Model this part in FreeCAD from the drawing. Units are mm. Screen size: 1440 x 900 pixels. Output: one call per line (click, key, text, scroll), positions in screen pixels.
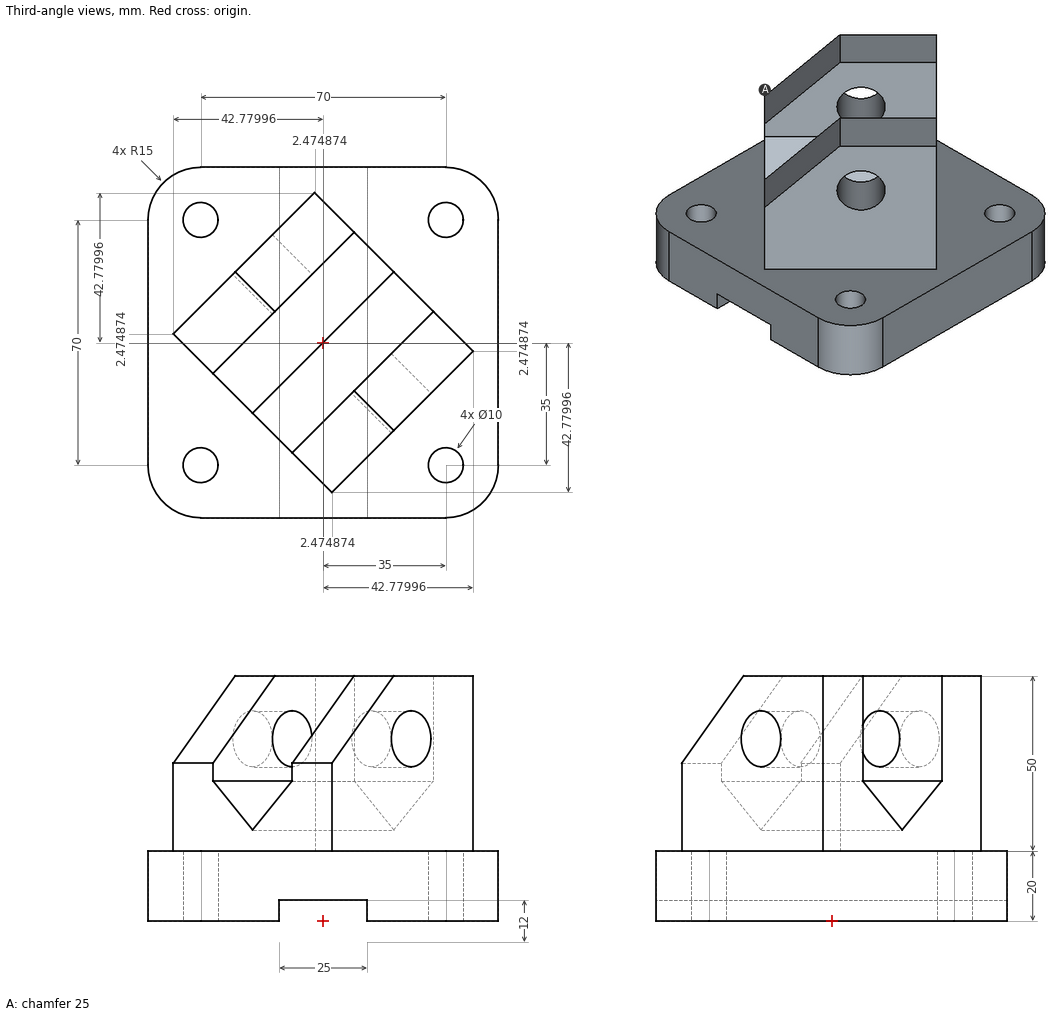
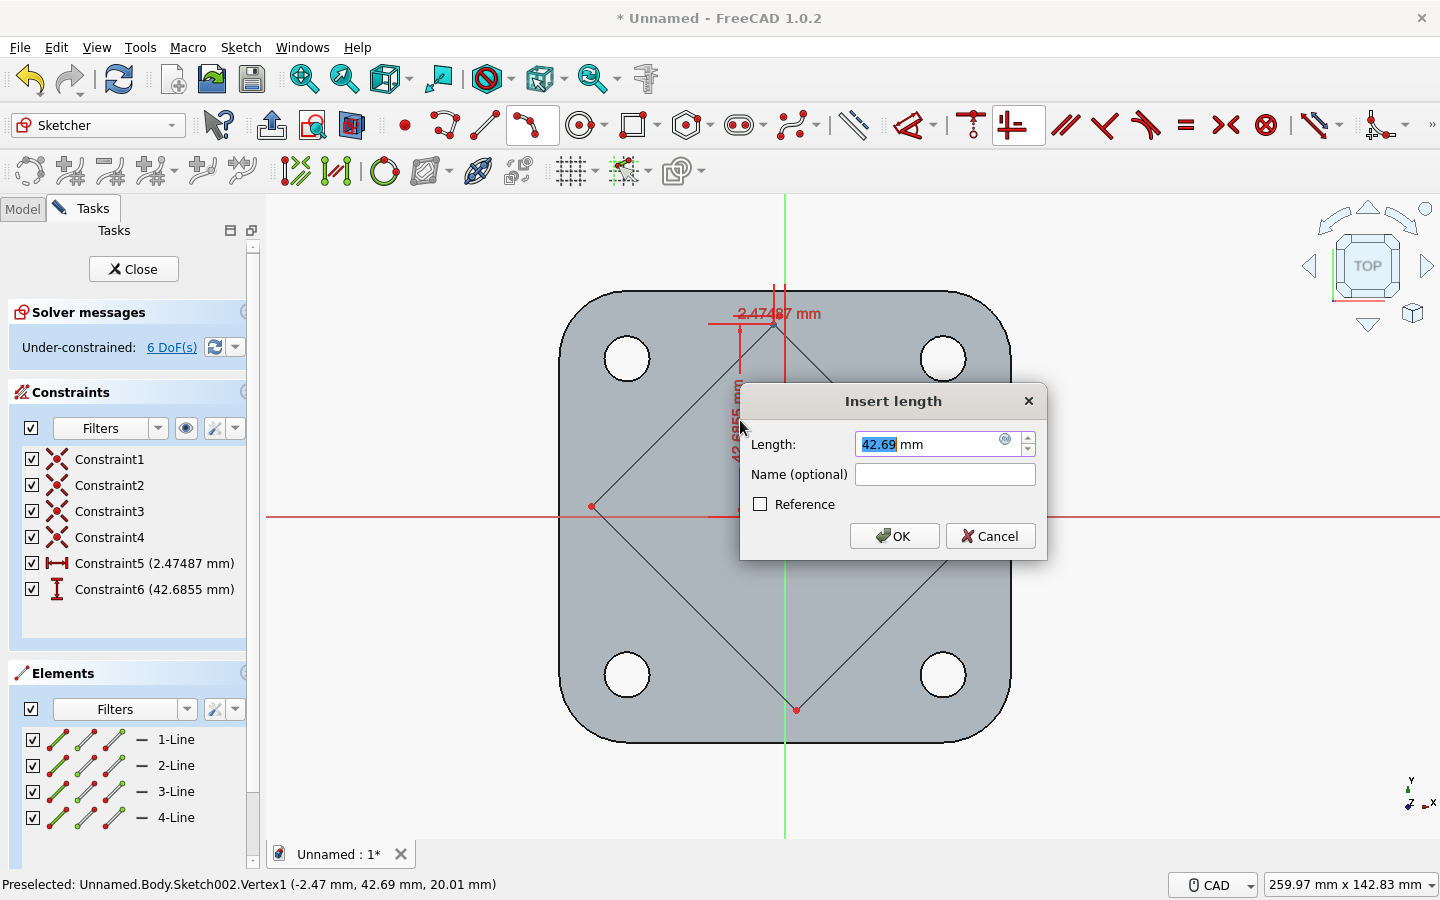
text(42.77996)
key(Return)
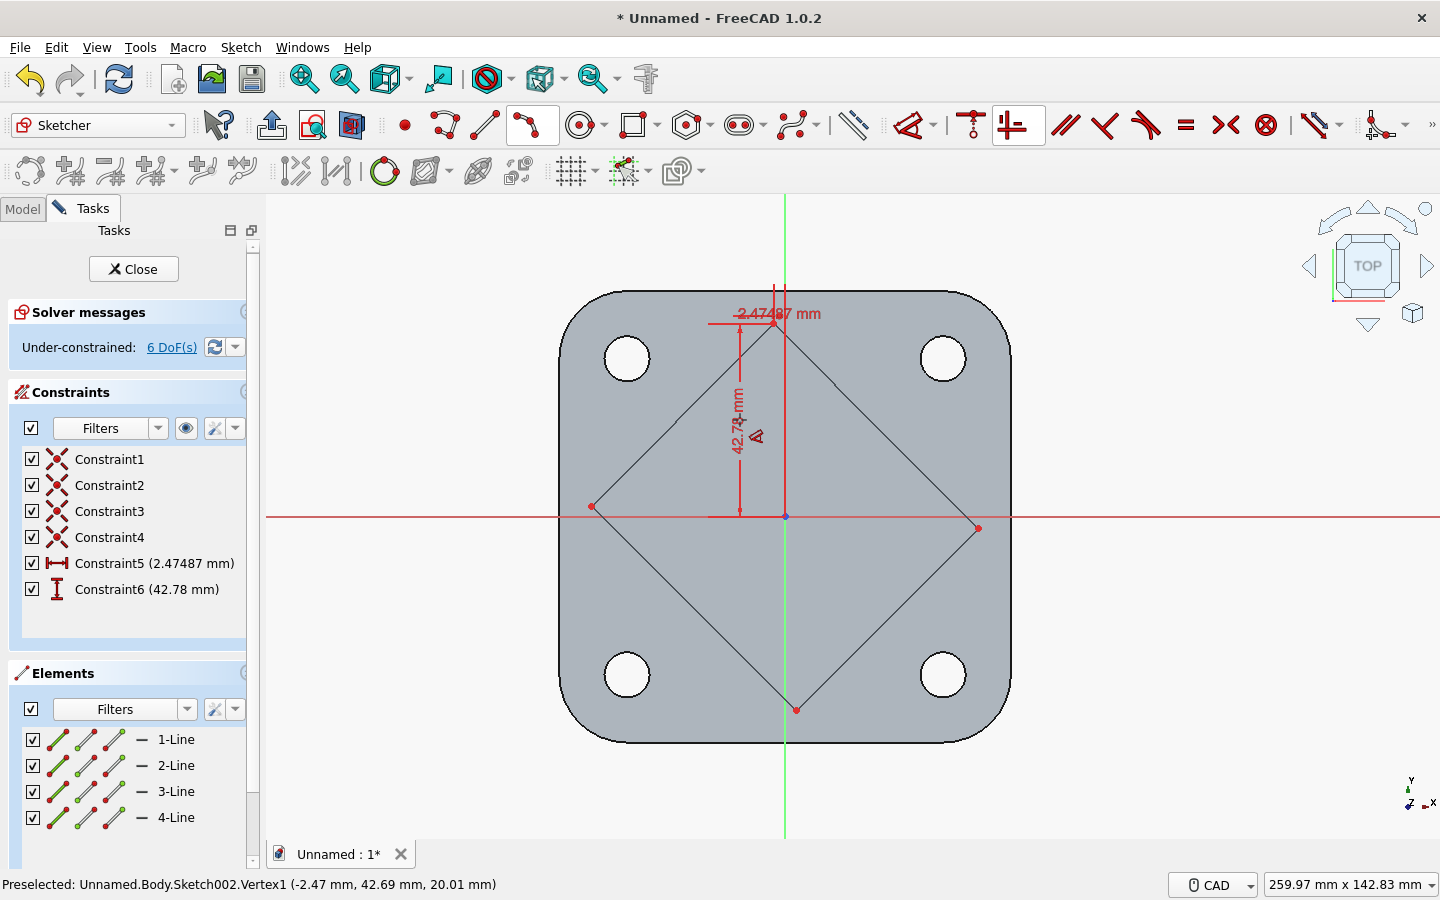
click(592, 506)
click(689, 472)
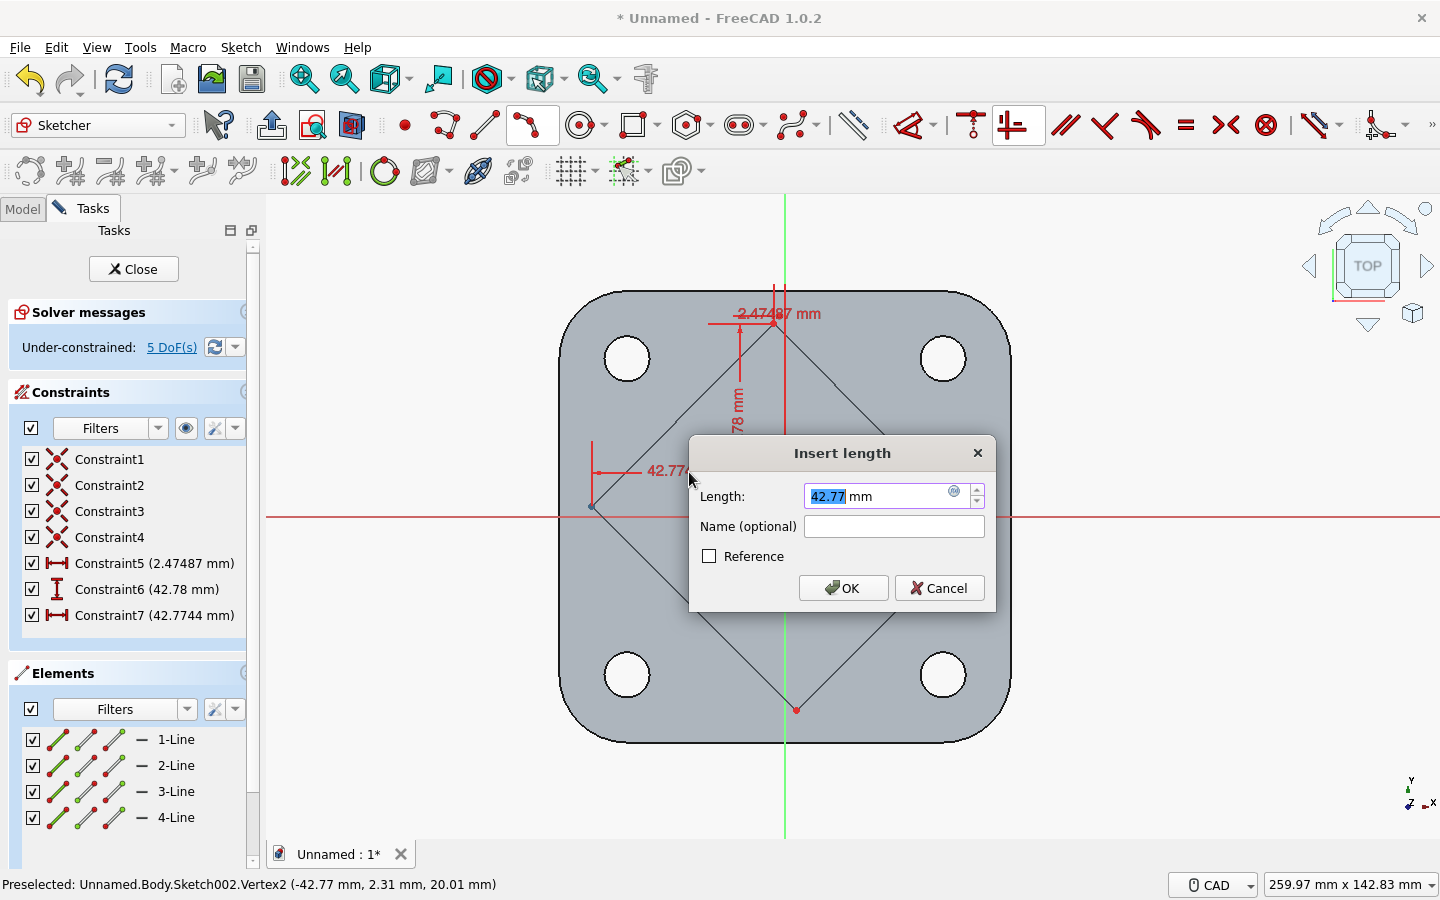
text(42.77996)
key(Return)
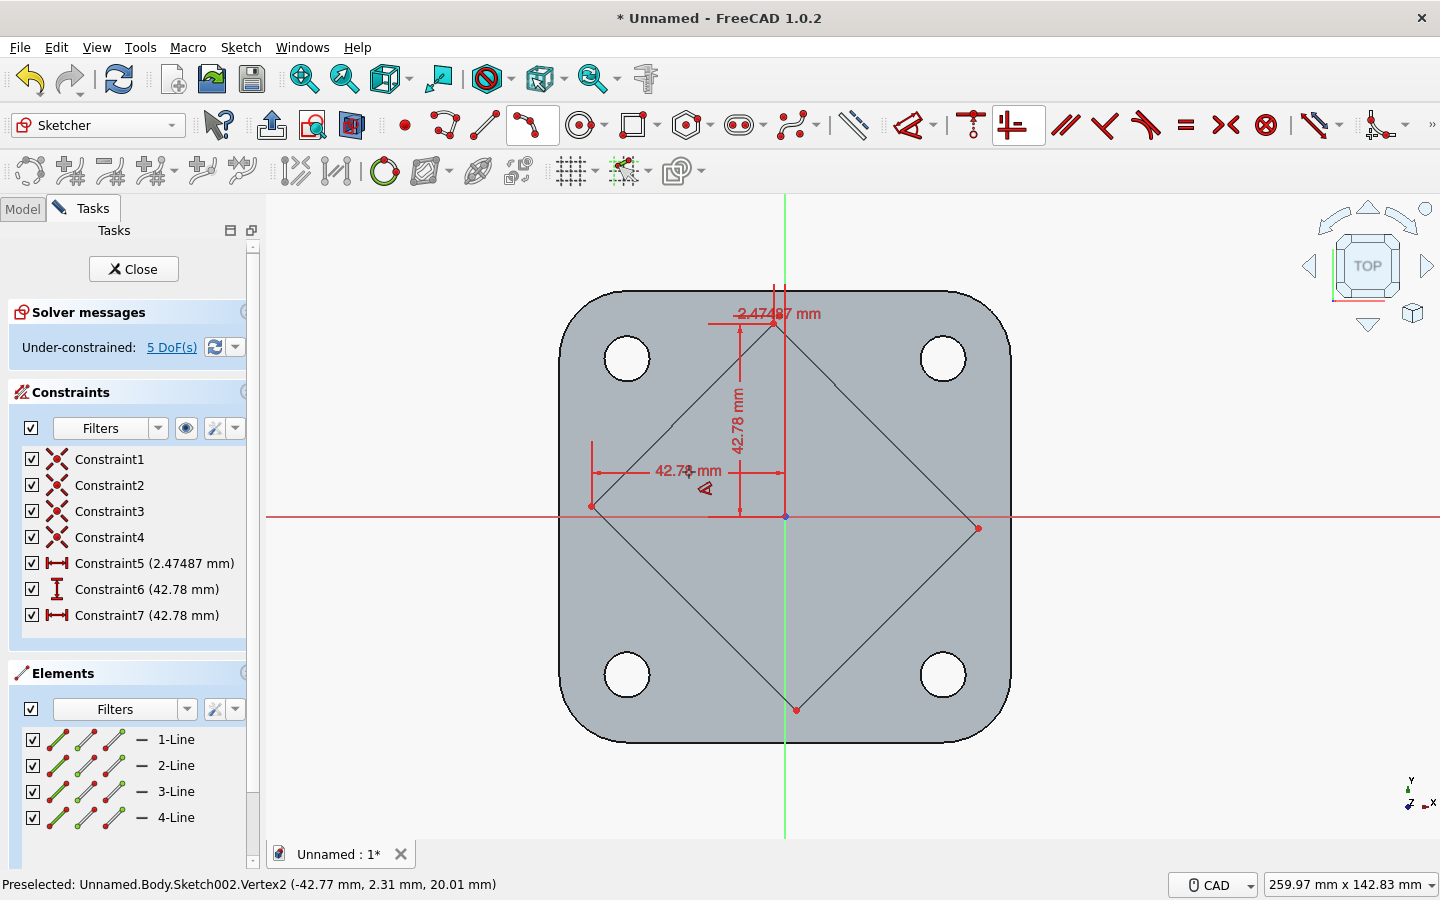
scroll(592, 506, up, 7)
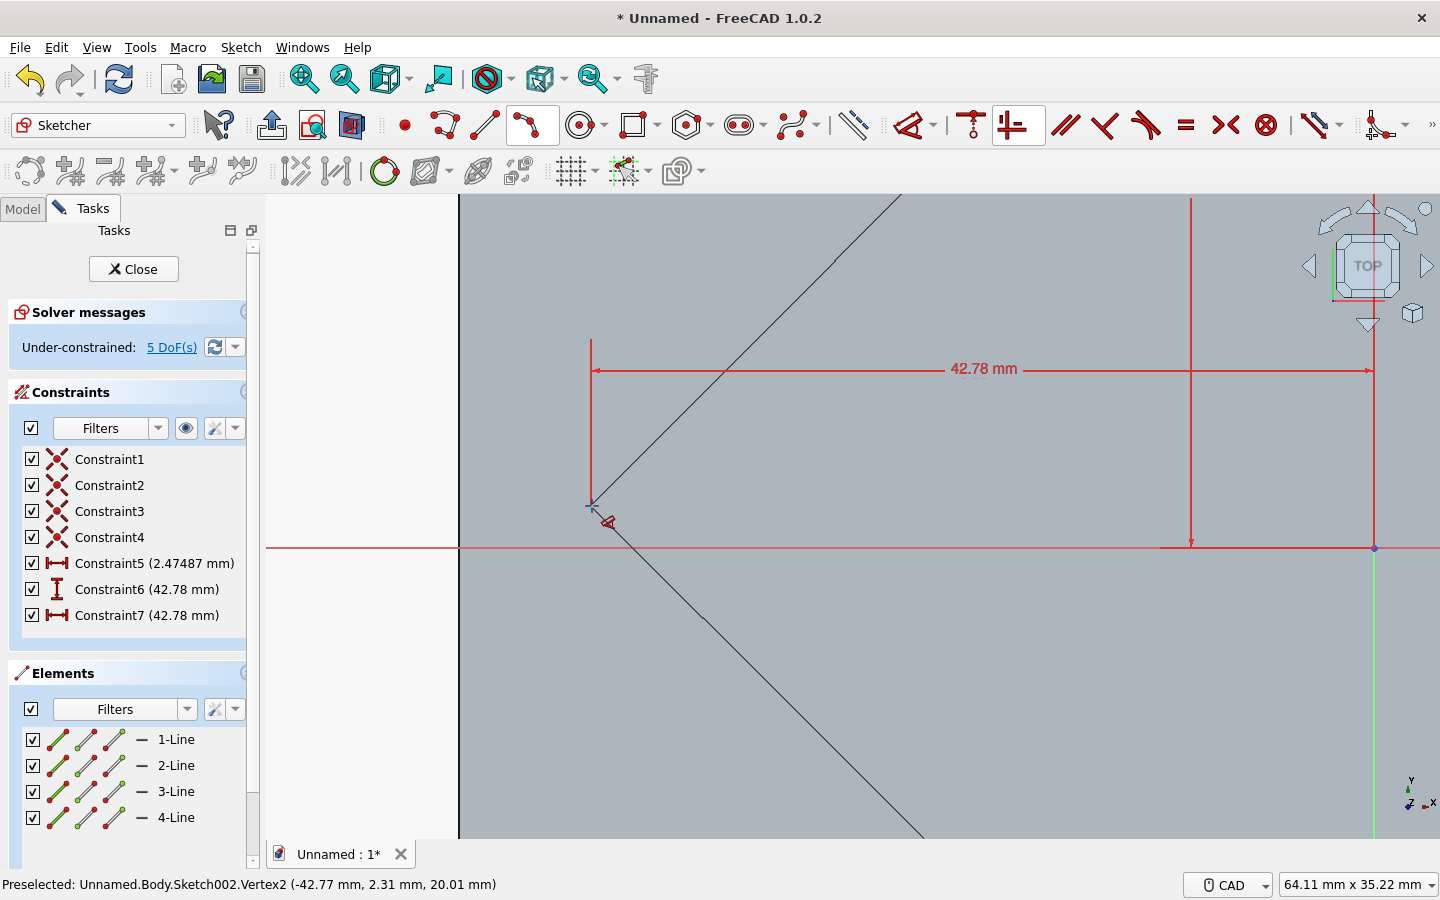
click(591, 506)
click(557, 527)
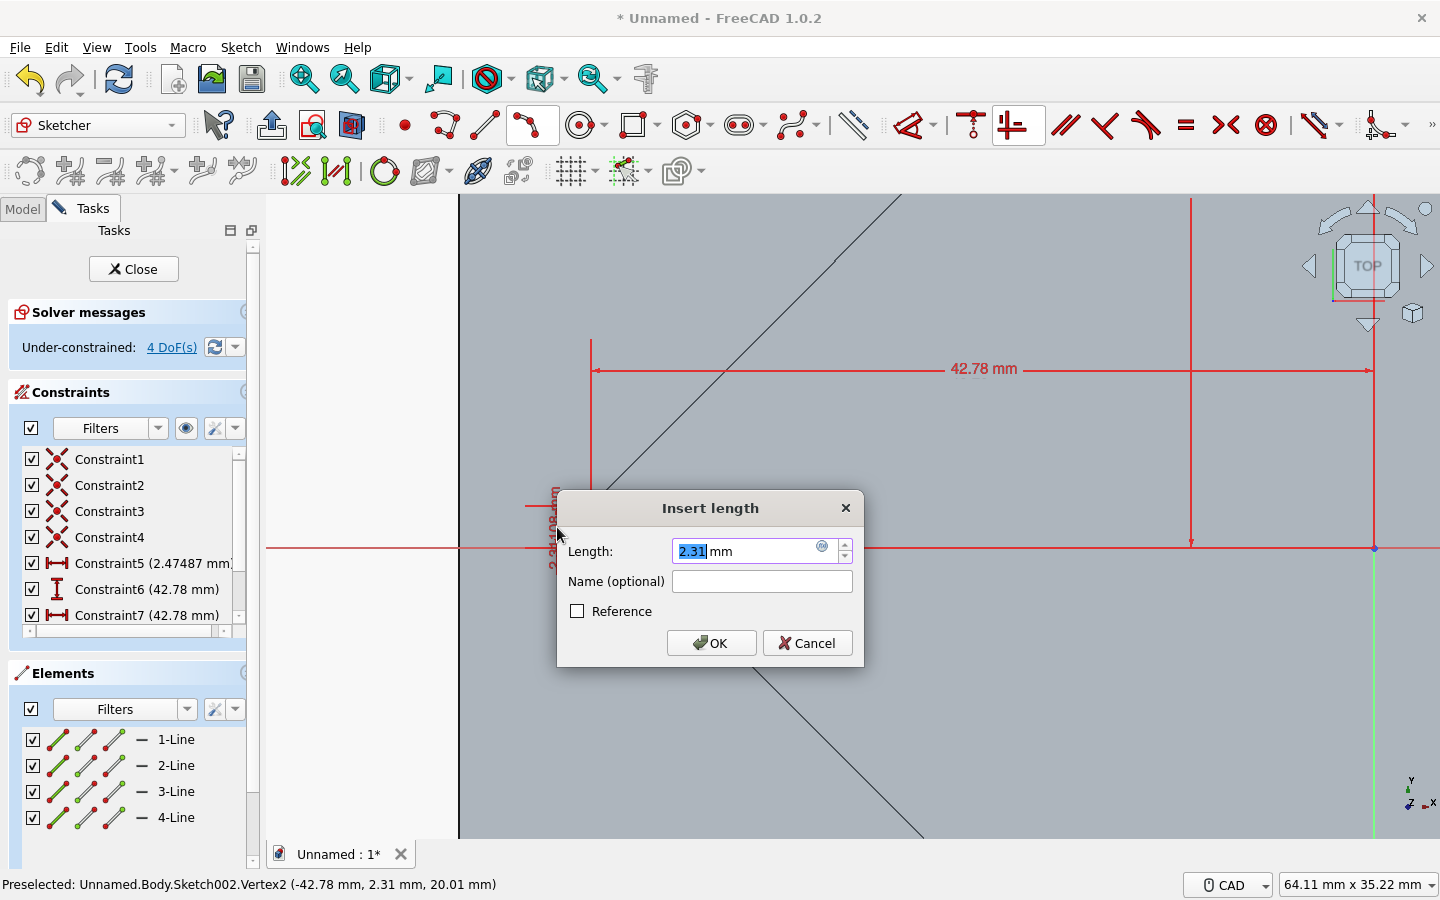
text(2.474874)
key(Return)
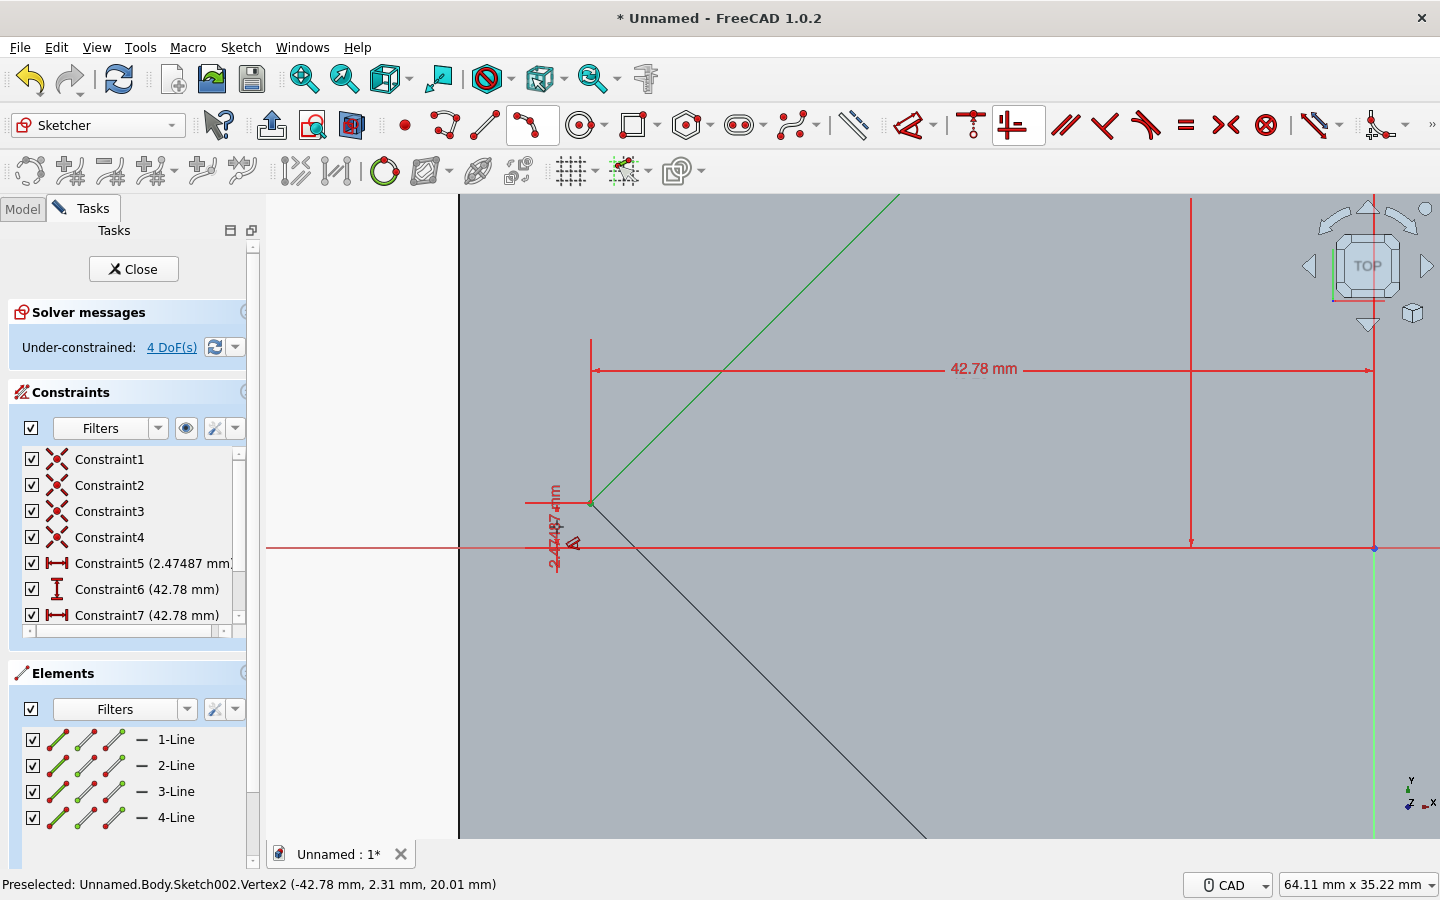
scroll(591, 506, down, 7)